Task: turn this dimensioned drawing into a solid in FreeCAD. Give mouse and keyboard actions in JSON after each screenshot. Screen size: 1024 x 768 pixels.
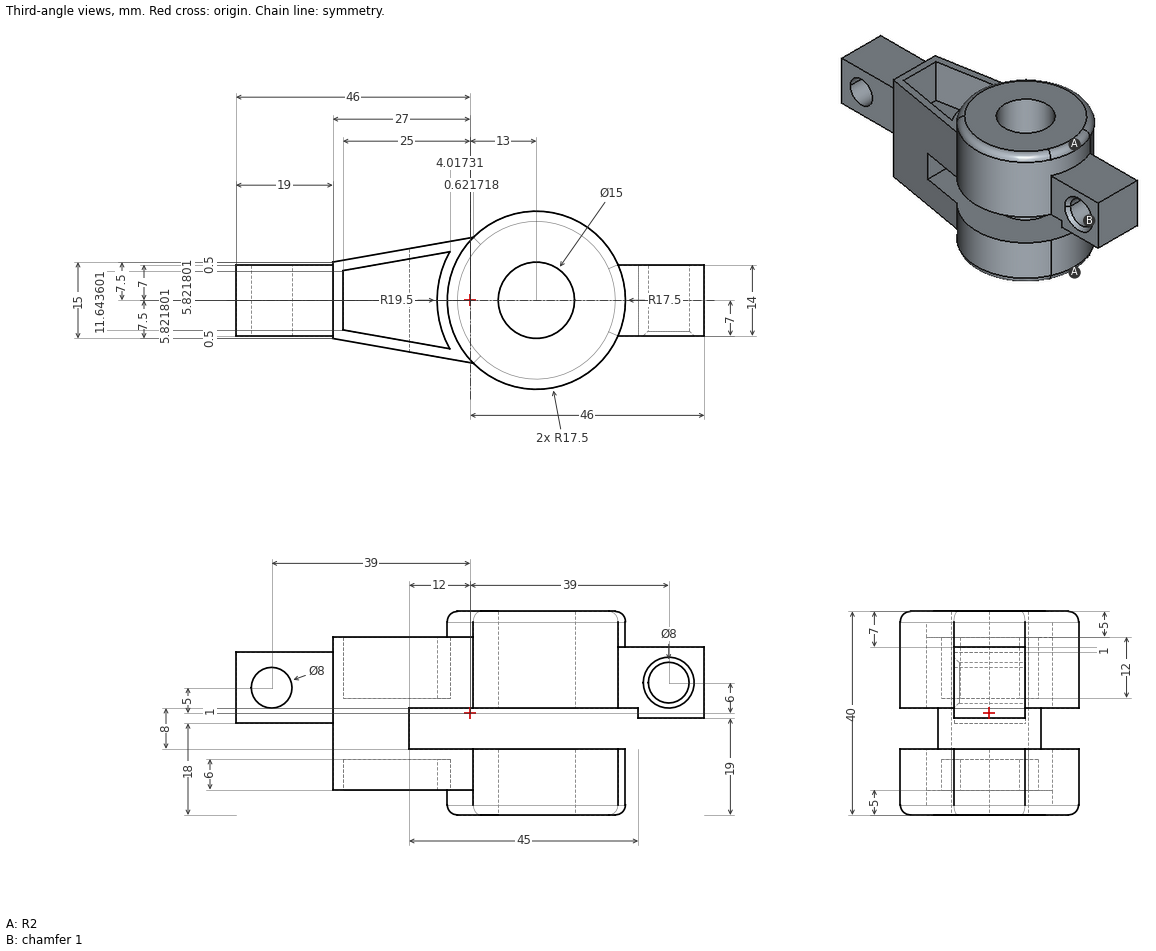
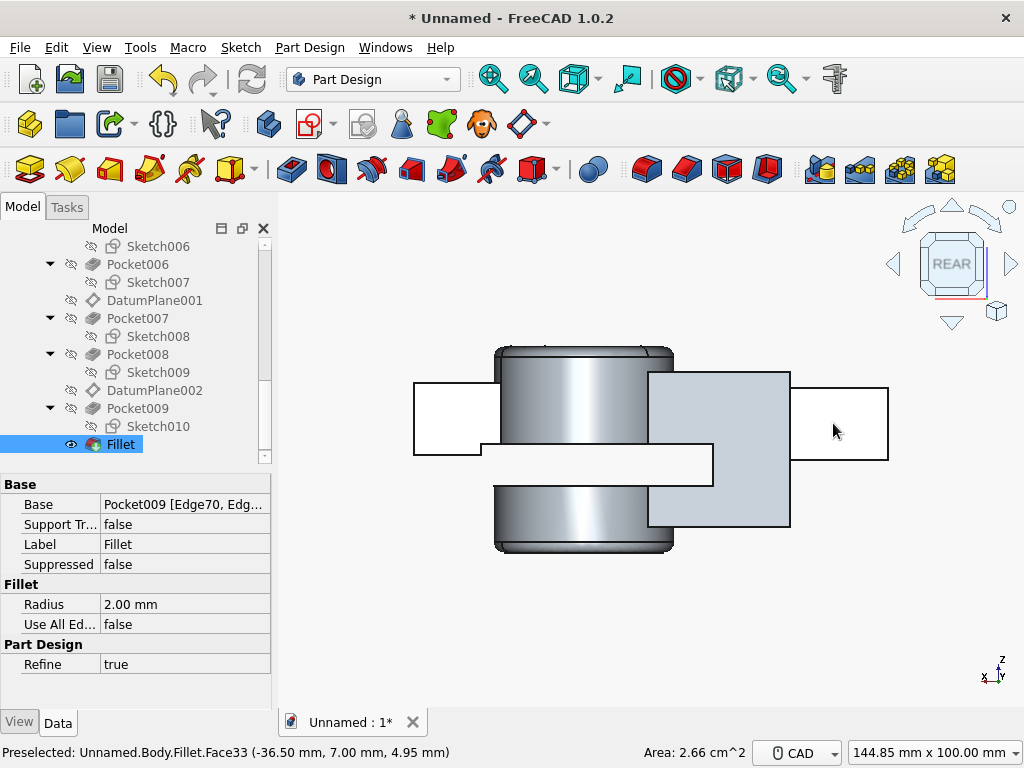
{"action": "left_click", "coordinate": [310, 124]}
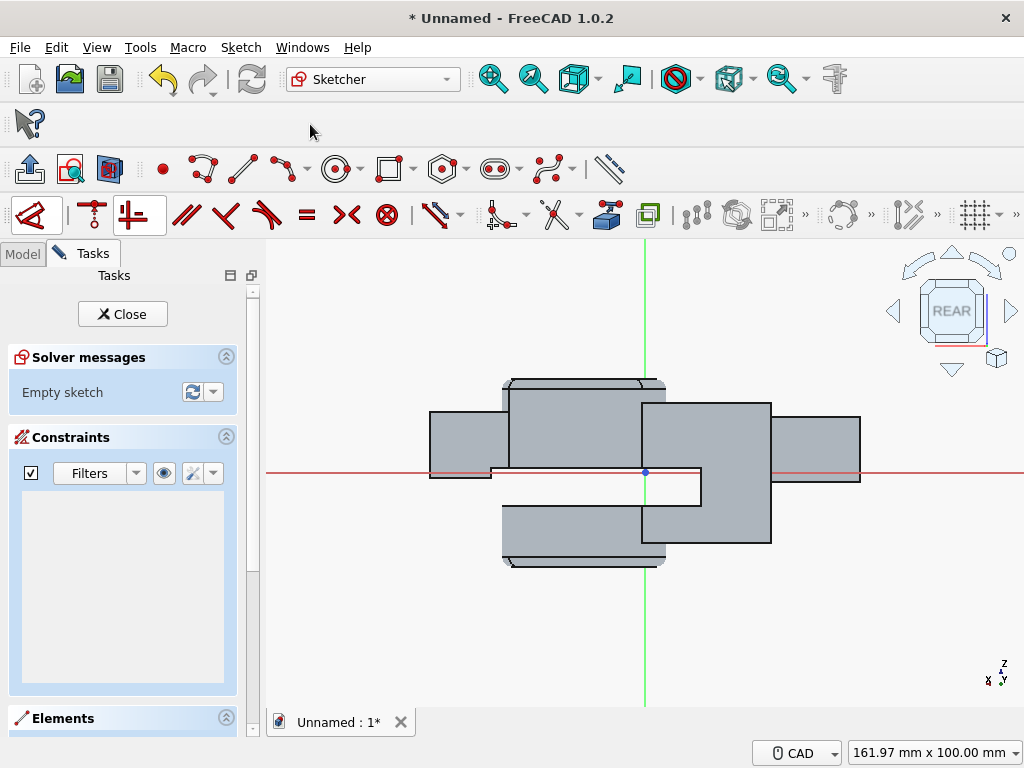
{"action": "scroll", "coordinate": [859, 446], "scroll_direction": "up", "scroll_amount": 10}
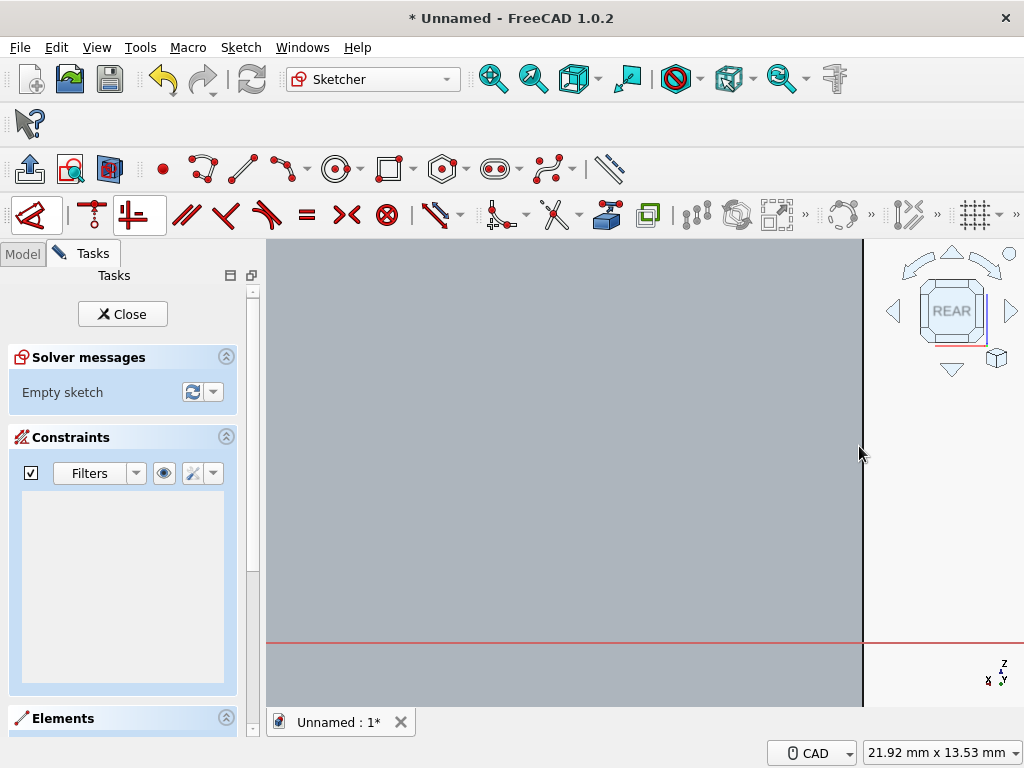
{"action": "left_click", "coordinate": [336, 170]}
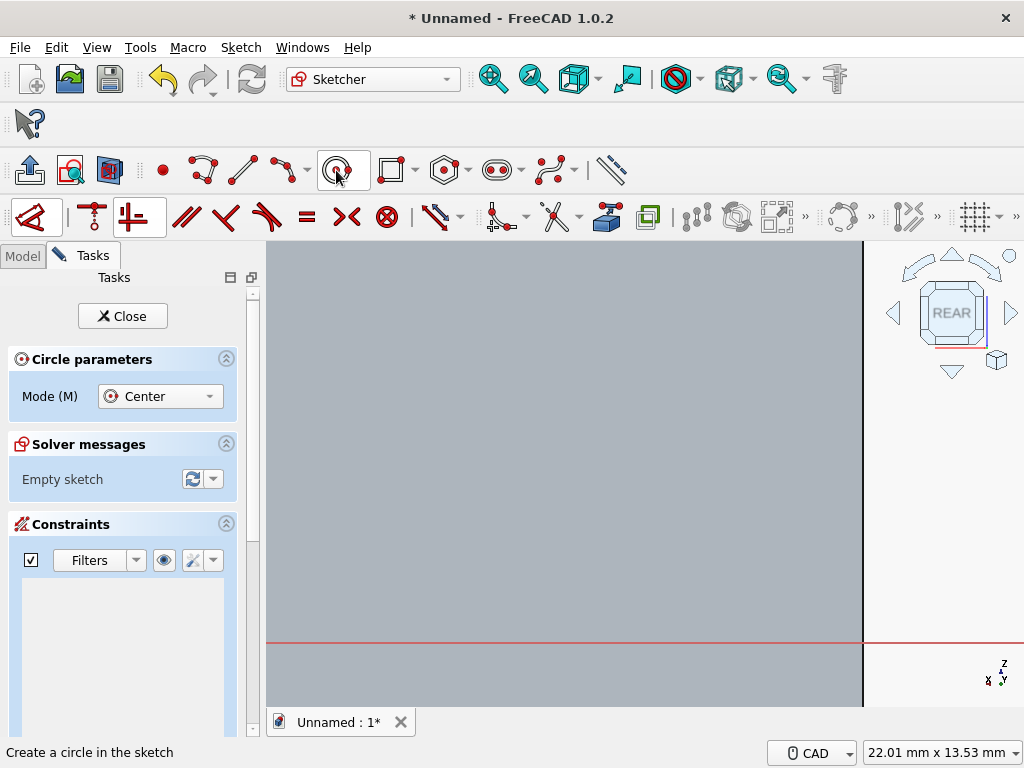
{"action": "left_click", "coordinate": [621, 471]}
{"action": "left_click", "coordinate": [719, 373]}
{"action": "key", "text": "Escape"}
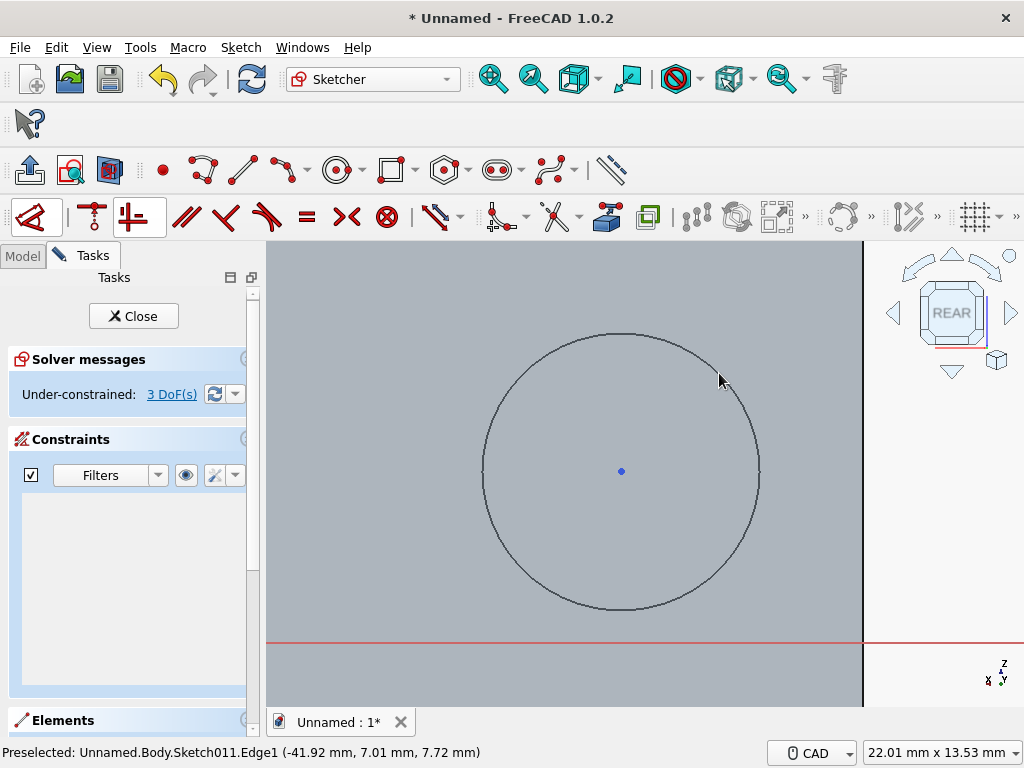
{"action": "left_click", "coordinate": [719, 374]}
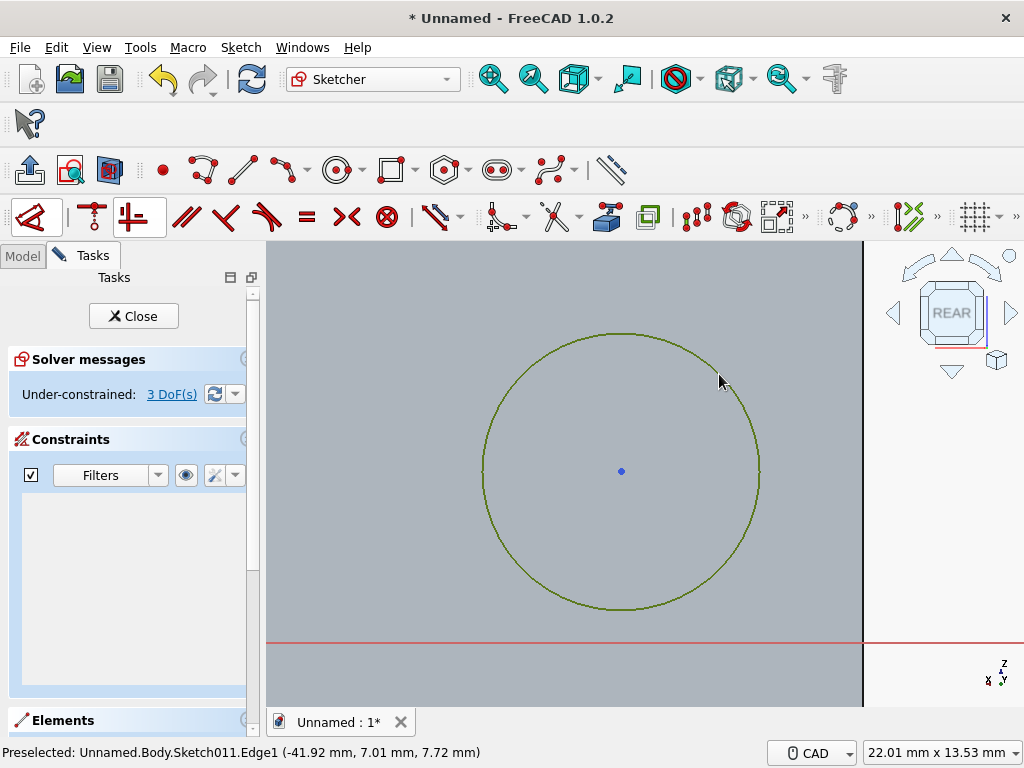
{"action": "key", "text": "k o"}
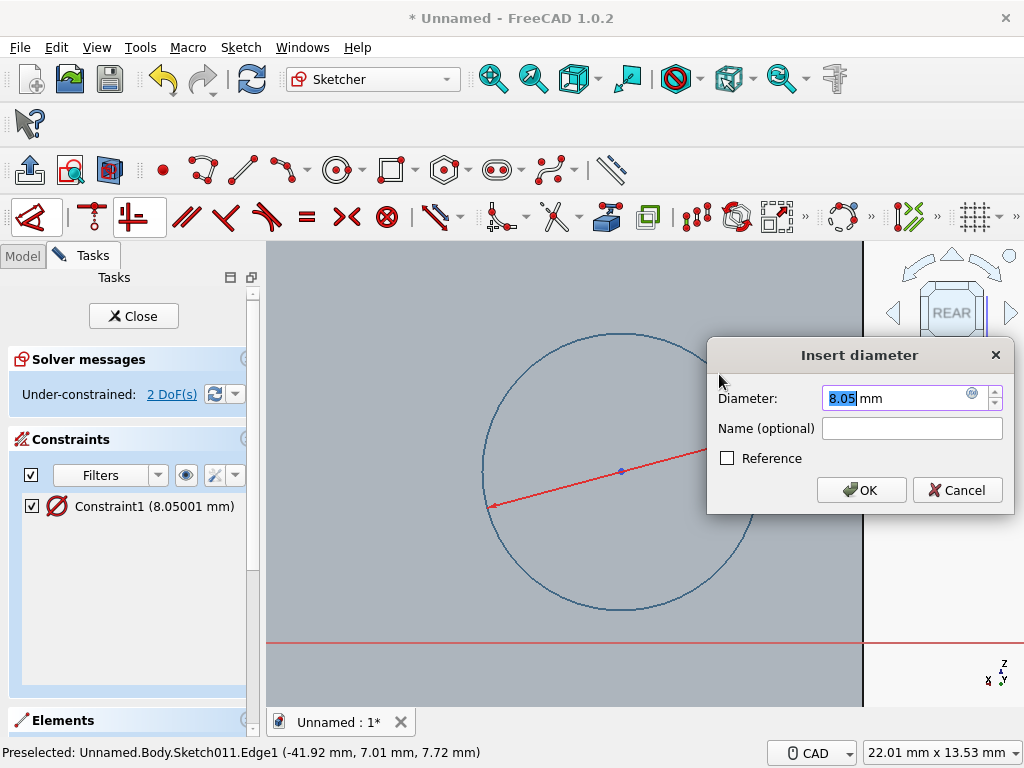
{"action": "type", "text": "8"}
{"action": "key", "text": "Return"}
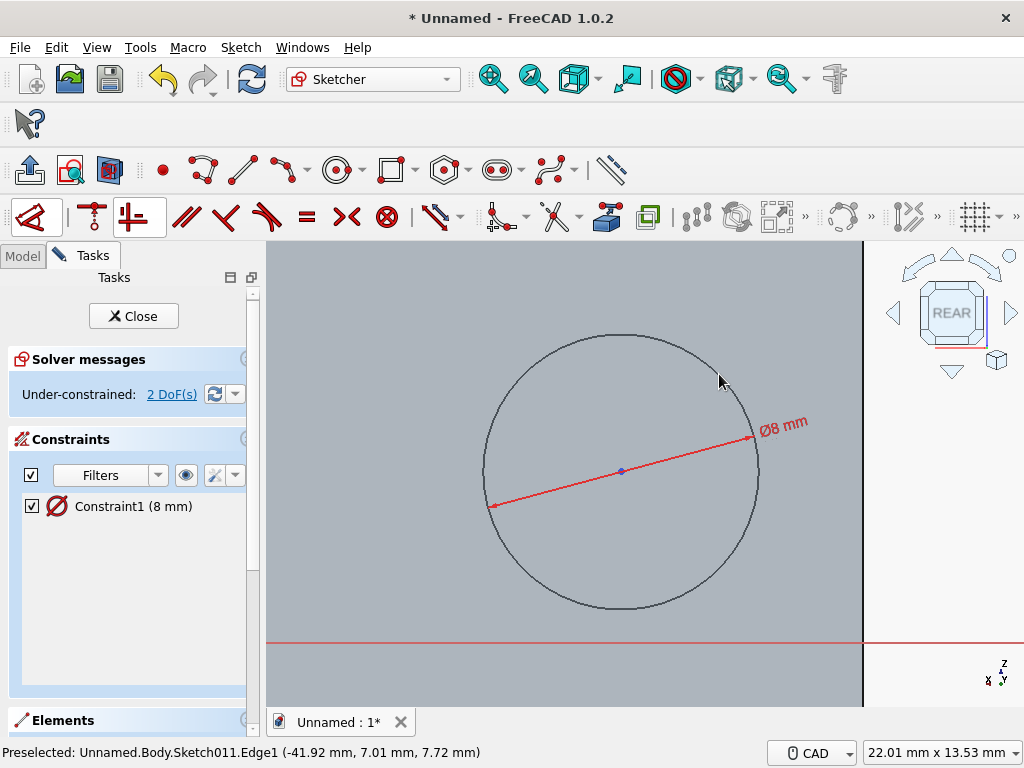
{"action": "left_click", "coordinate": [621, 472]}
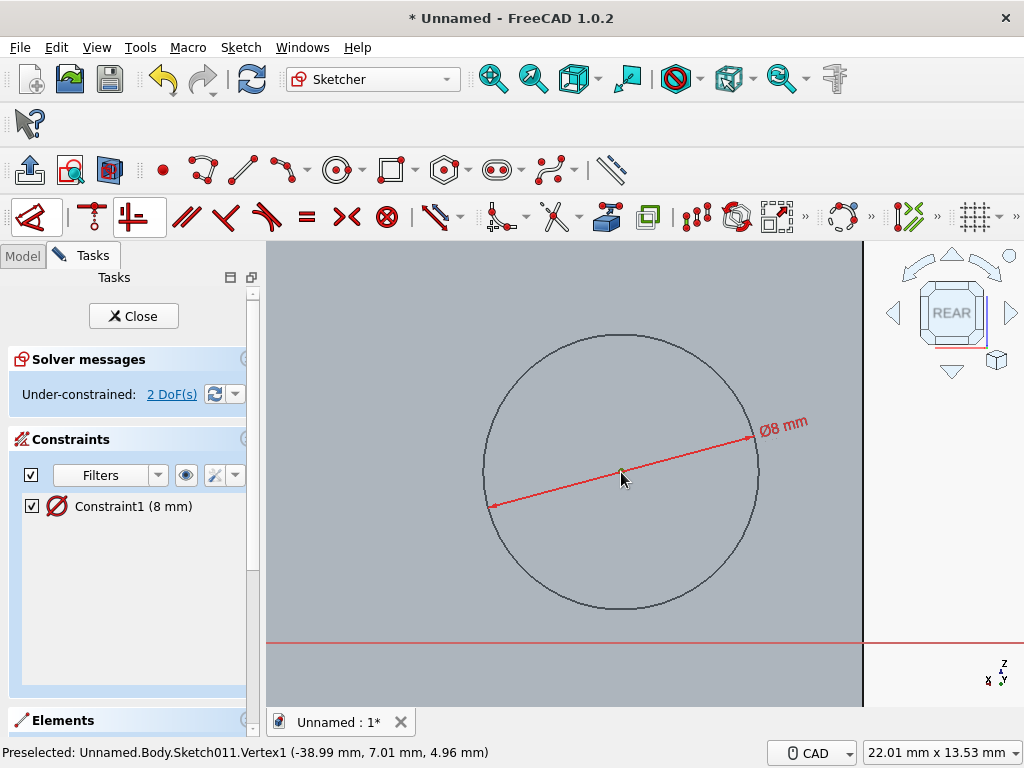
{"action": "left_click", "coordinate": [56, 218]}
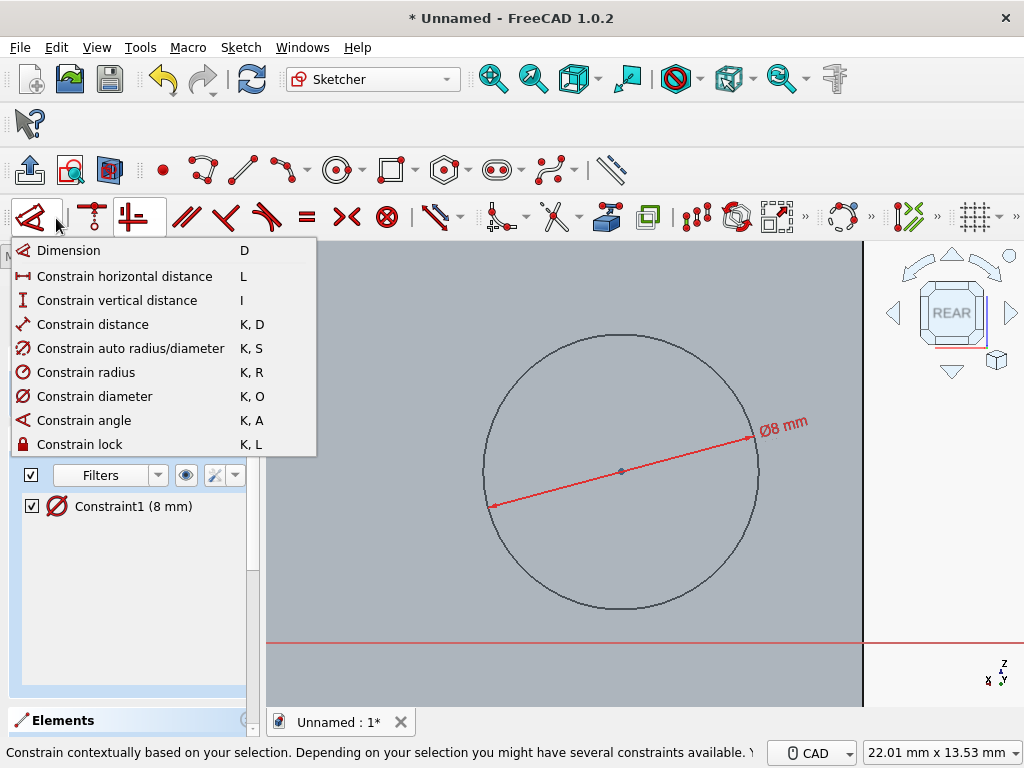
{"action": "left_click", "coordinate": [164, 300]}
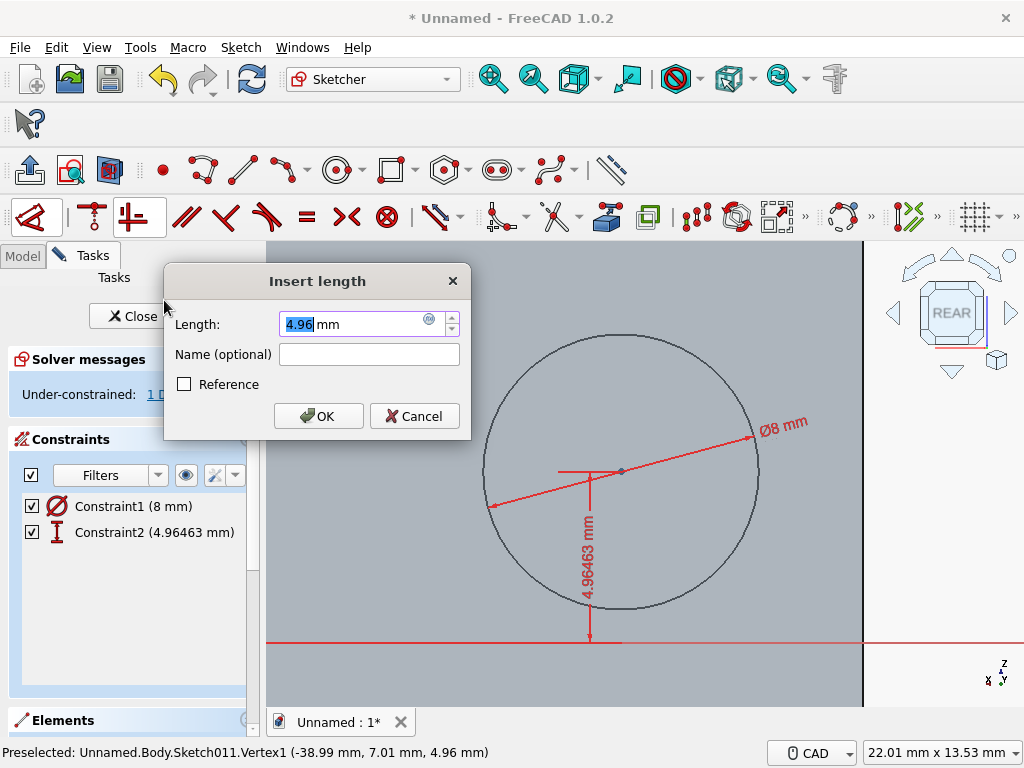
{"action": "type", "text": "5"}
{"action": "key", "text": "Return"}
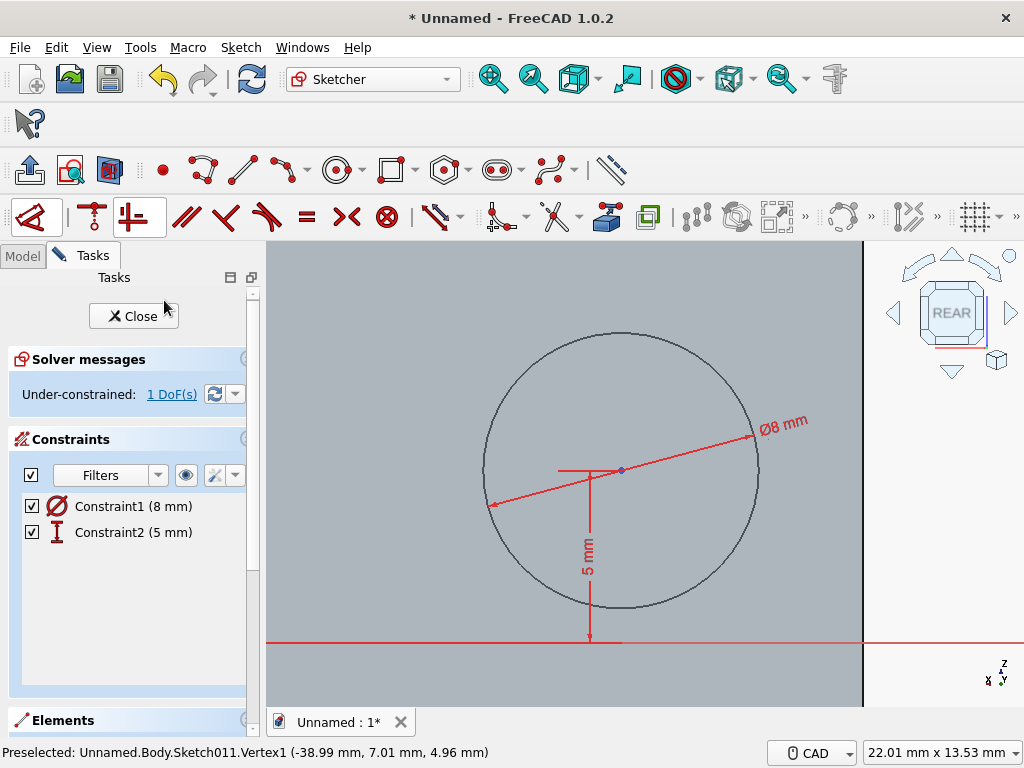
{"action": "left_click", "coordinate": [621, 471]}